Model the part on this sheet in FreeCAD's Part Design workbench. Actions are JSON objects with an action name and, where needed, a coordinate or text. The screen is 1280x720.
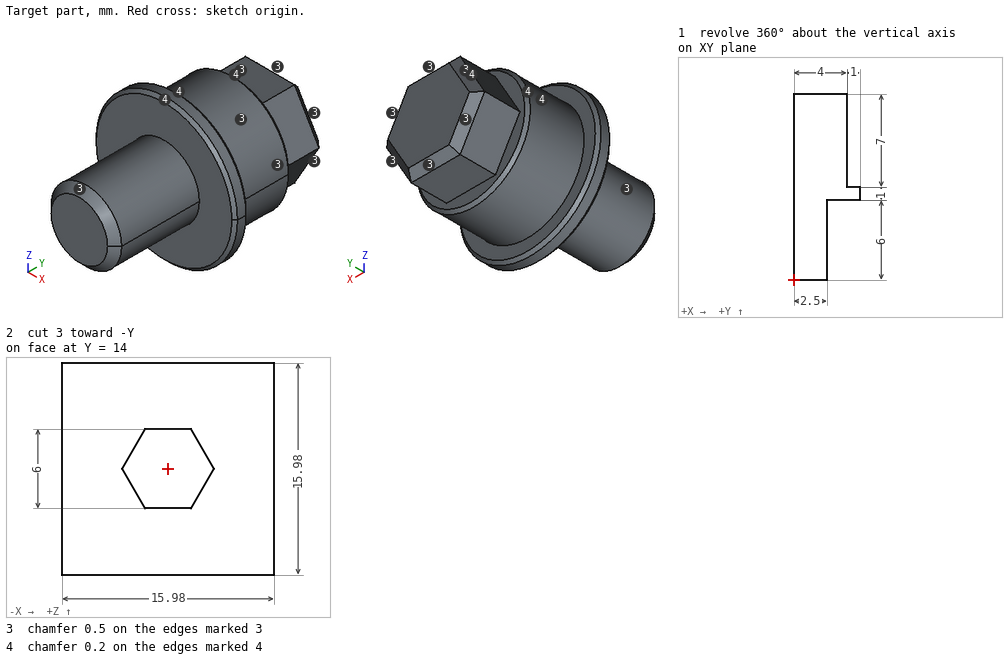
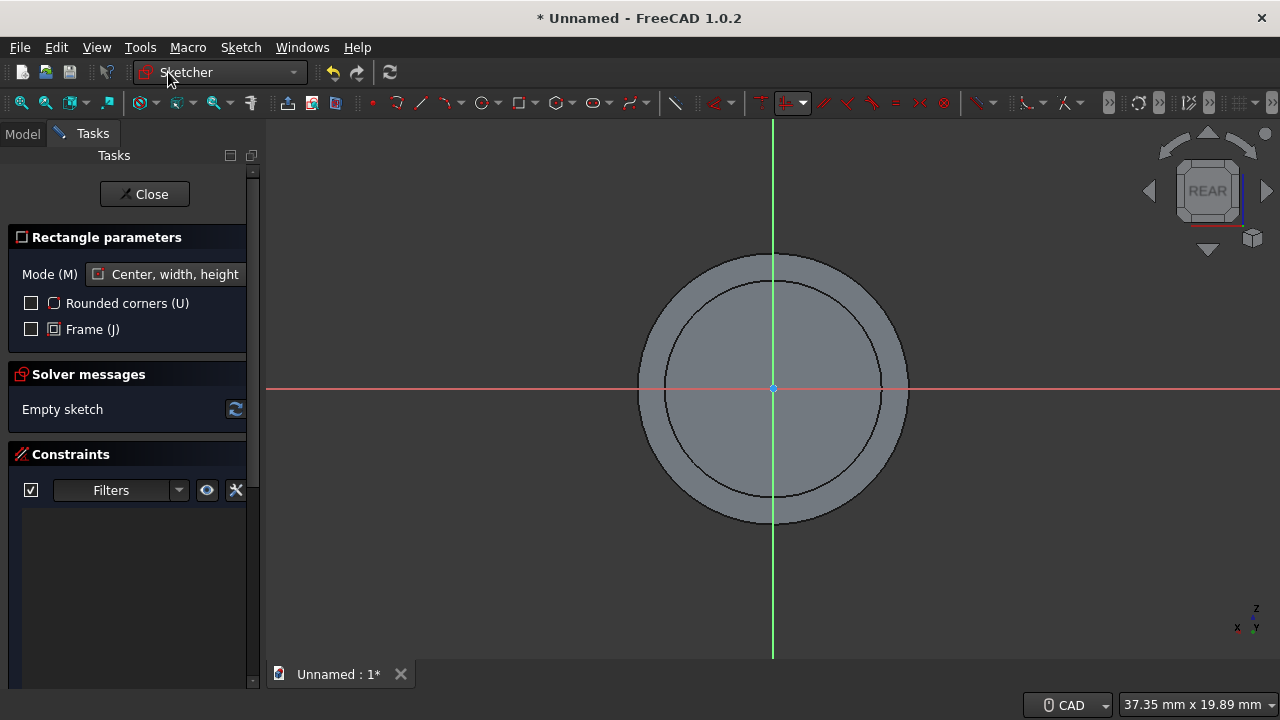
{"action": "left_click", "coordinate": [773, 389]}
{"action": "left_click", "coordinate": [990, 172]}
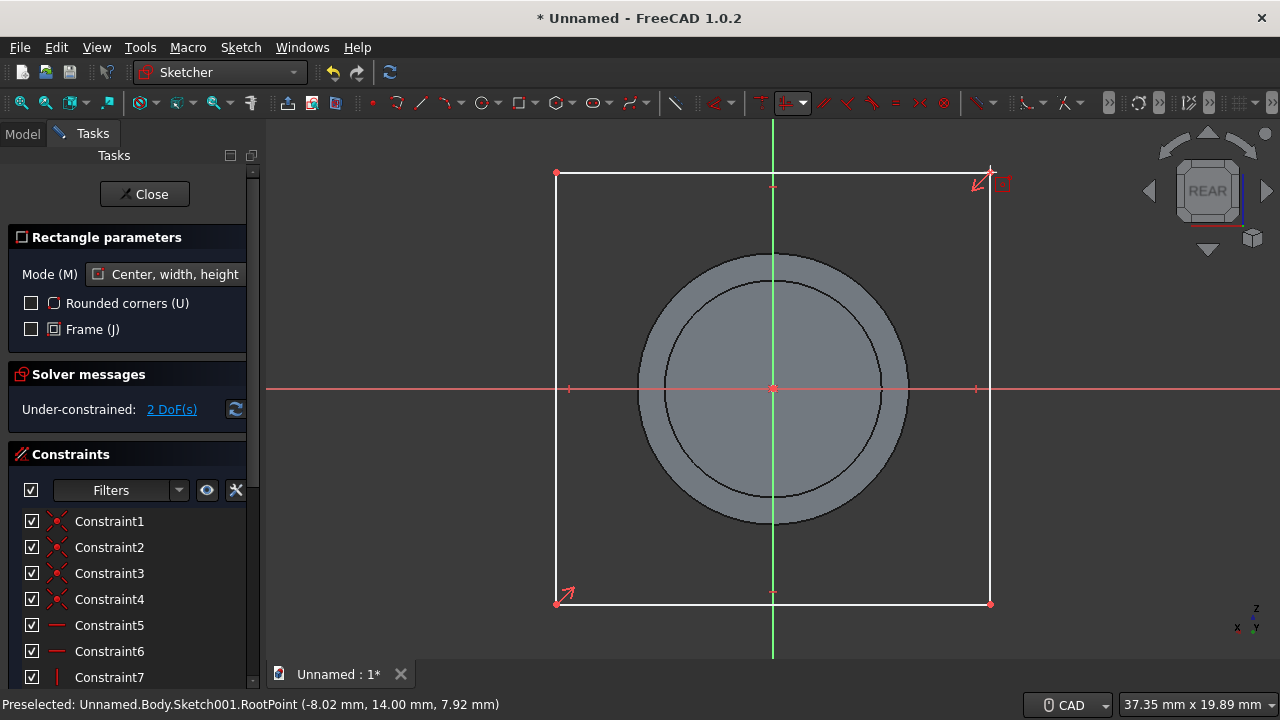
{"action": "left_click", "coordinate": [556, 104]}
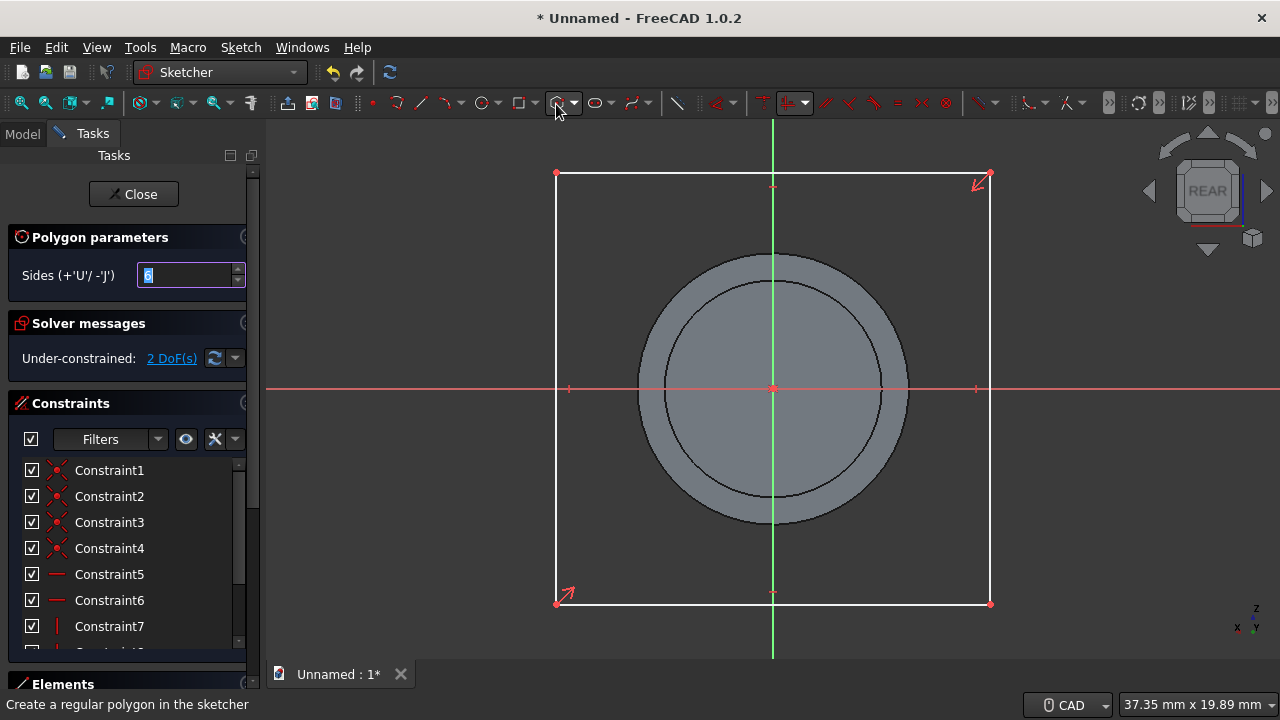
{"action": "left_click", "coordinate": [773, 389]}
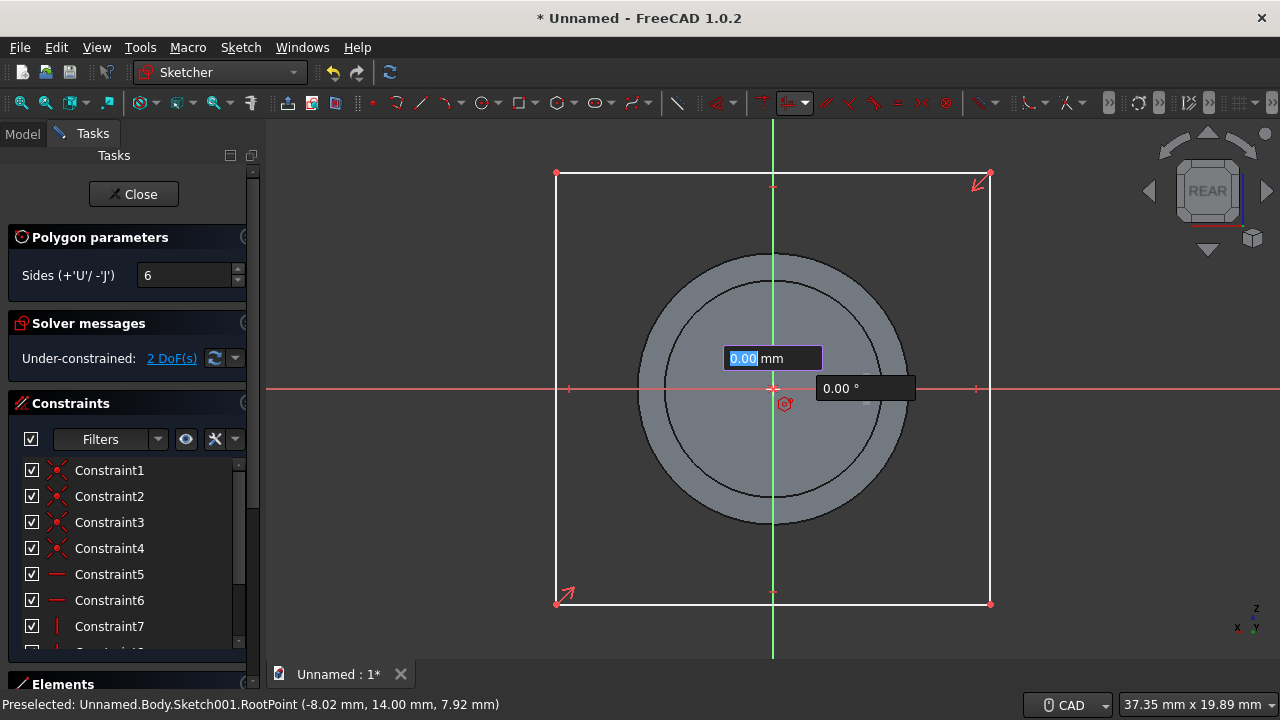
{"action": "left_click", "coordinate": [679, 389]}
{"action": "key", "text": "Escape"}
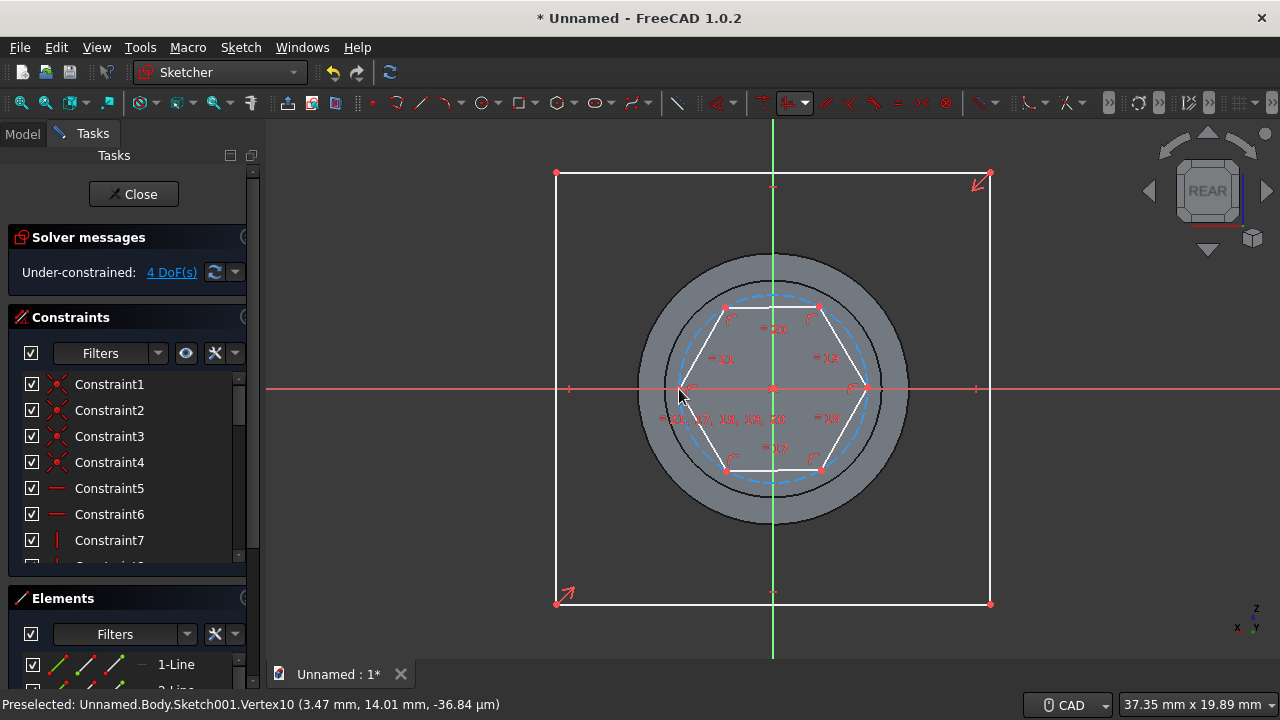
{"action": "scroll", "coordinate": [755, 471], "scroll_direction": "up", "scroll_amount": 2}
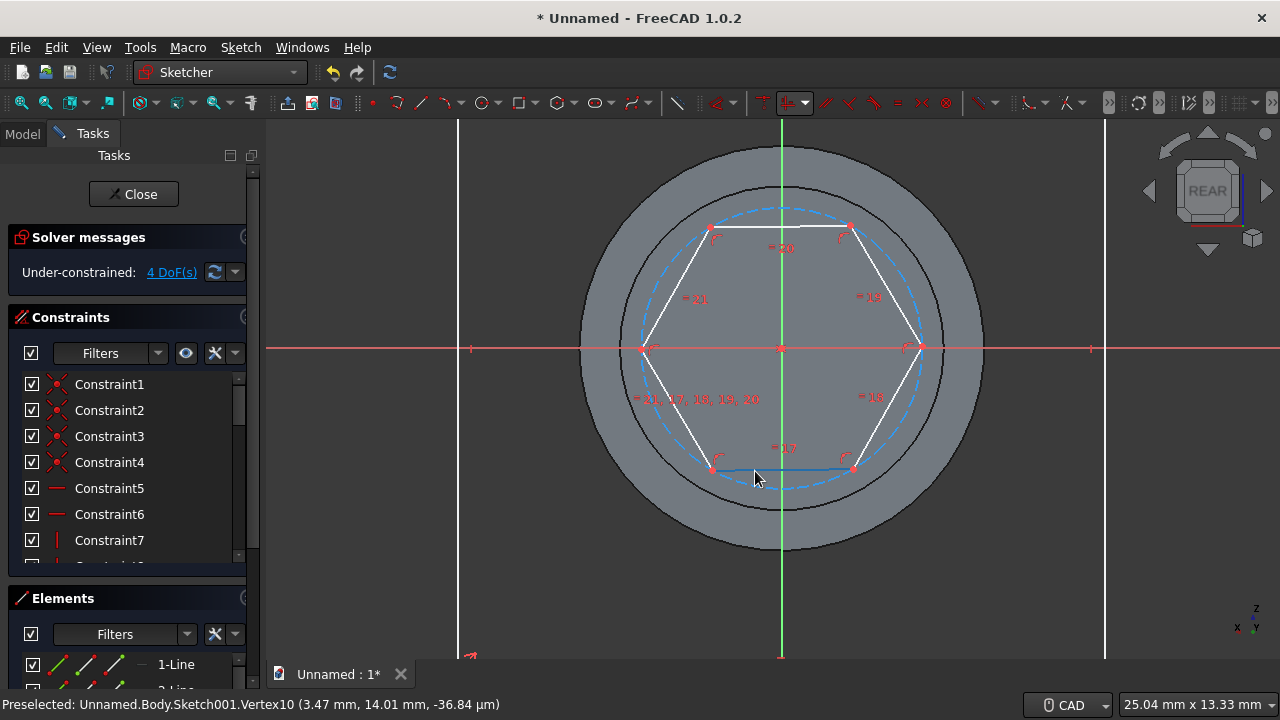
{"action": "left_click", "coordinate": [755, 470]}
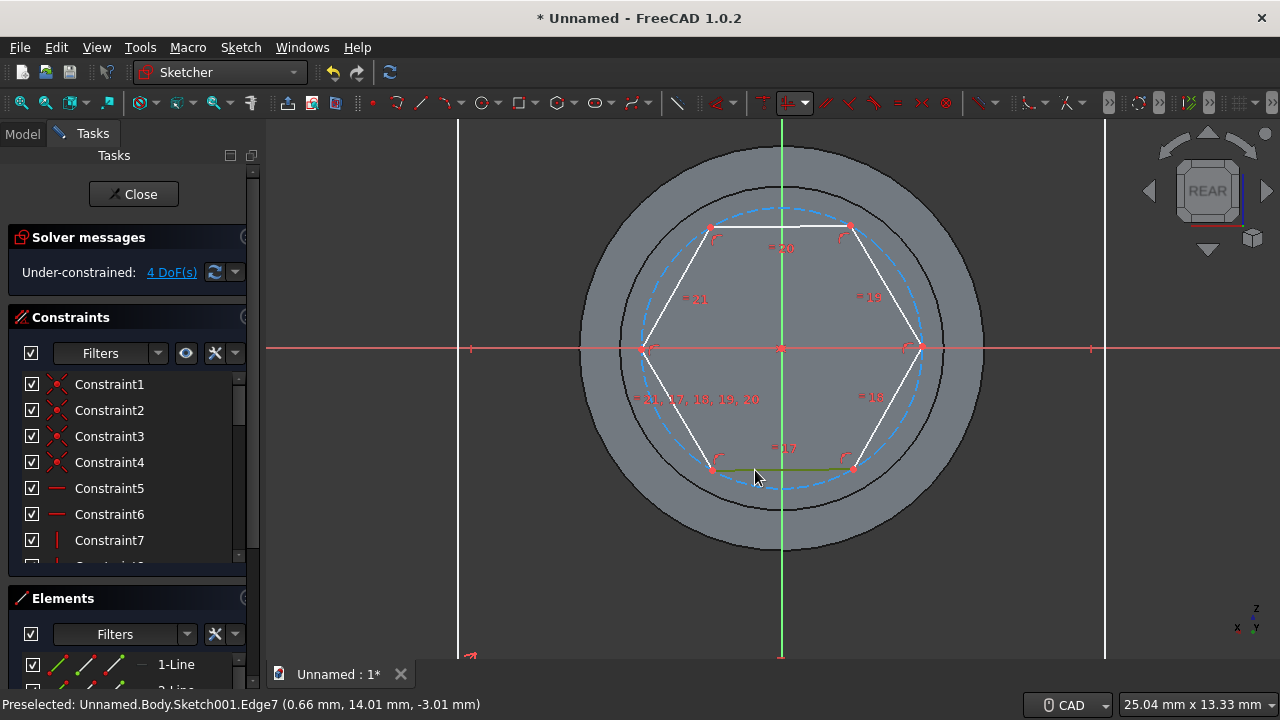
{"action": "left_click", "coordinate": [808, 104]}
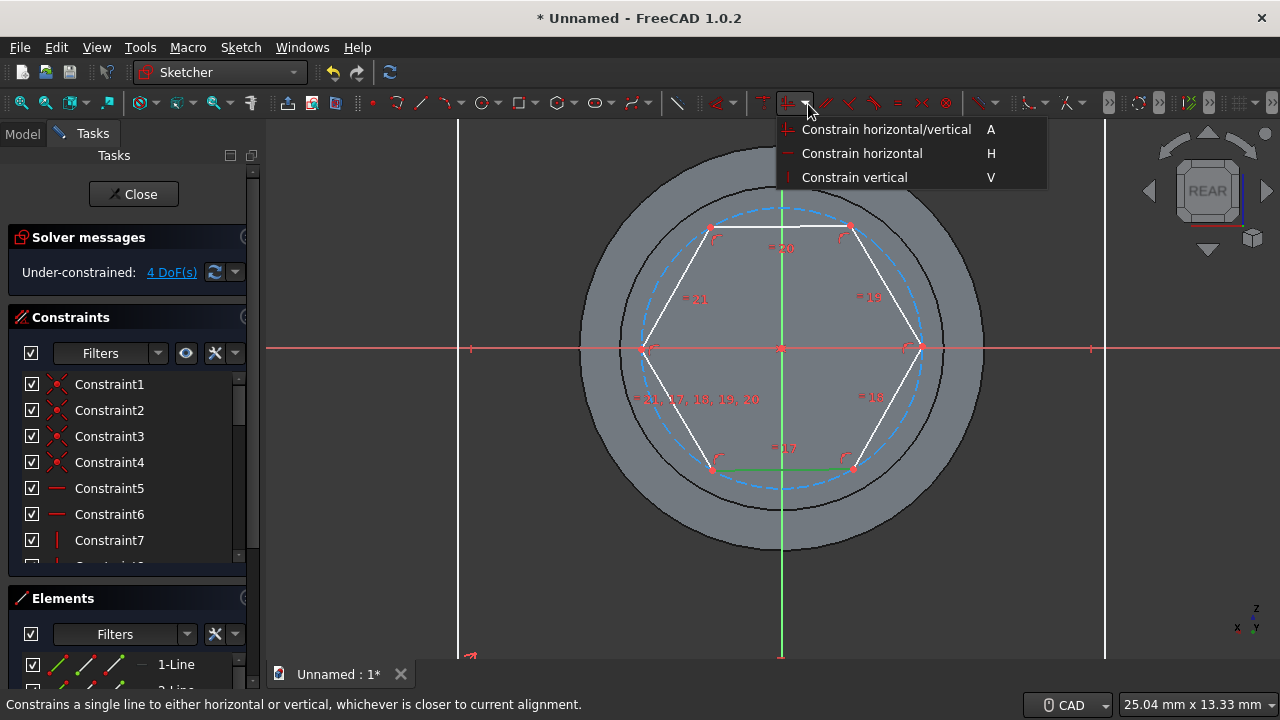
{"action": "left_click", "coordinate": [912, 153]}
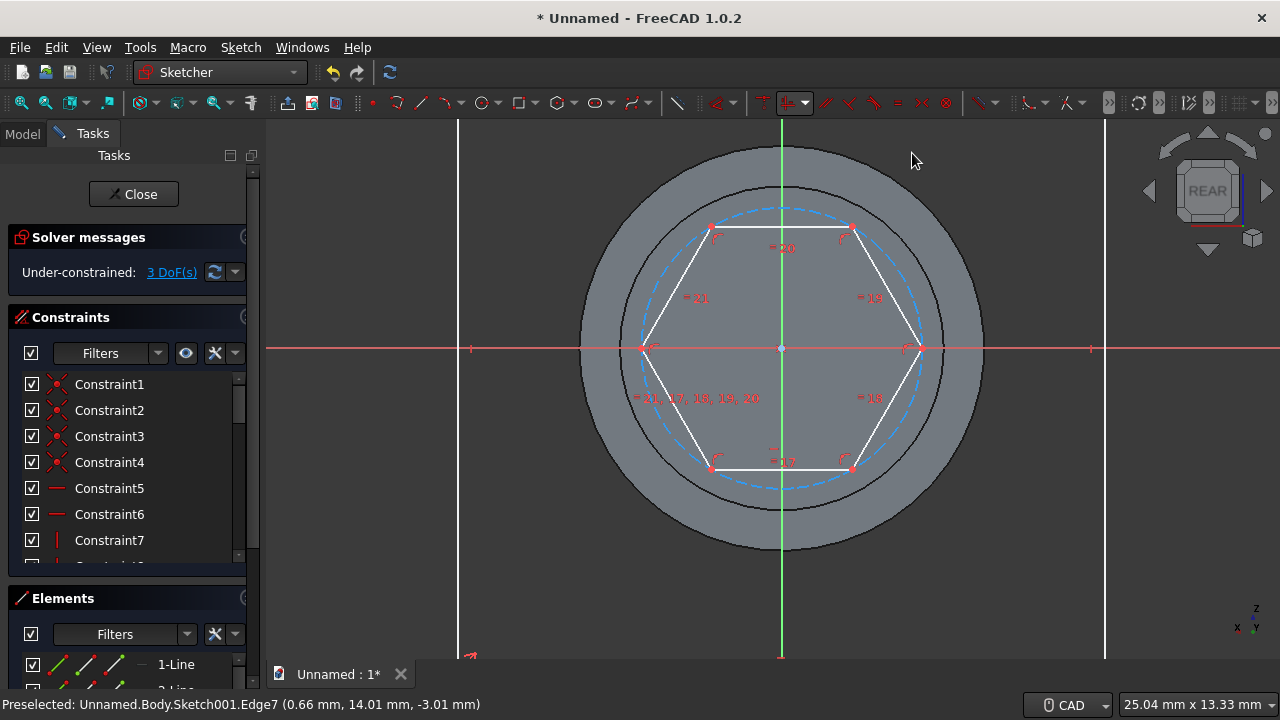
{"action": "left_click", "coordinate": [716, 104]}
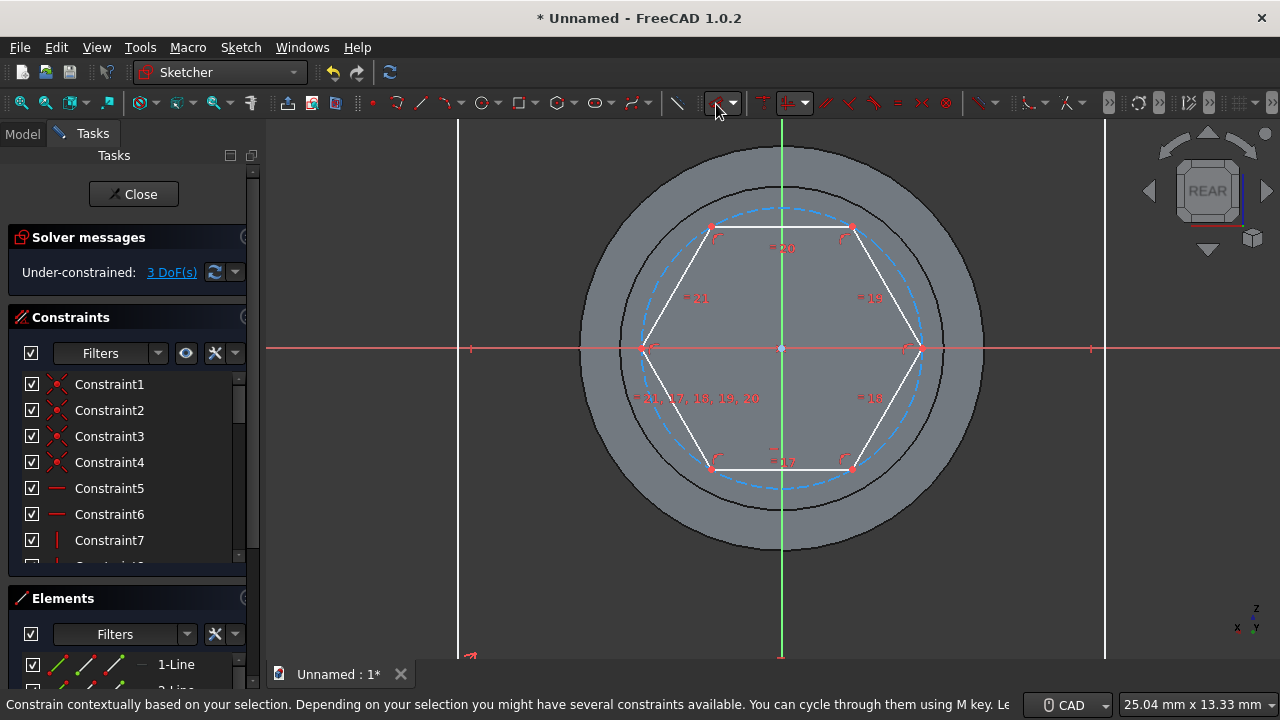
{"action": "left_click", "coordinate": [712, 470]}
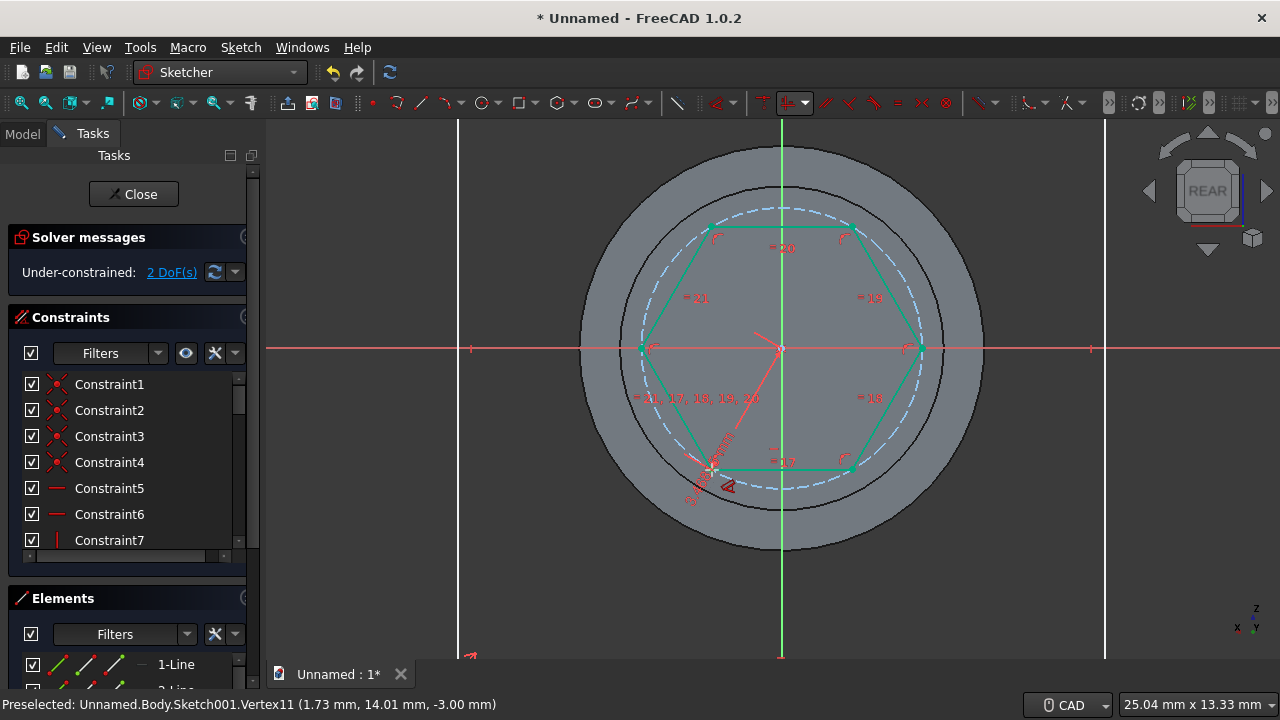
{"action": "left_click", "coordinate": [852, 227]}
{"action": "left_click", "coordinate": [910, 263]}